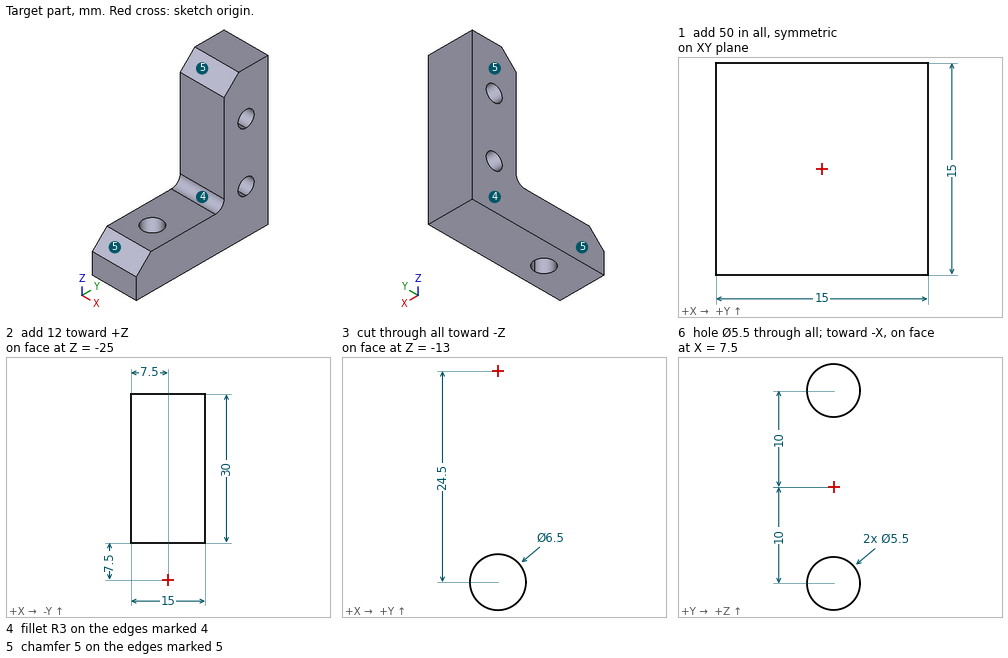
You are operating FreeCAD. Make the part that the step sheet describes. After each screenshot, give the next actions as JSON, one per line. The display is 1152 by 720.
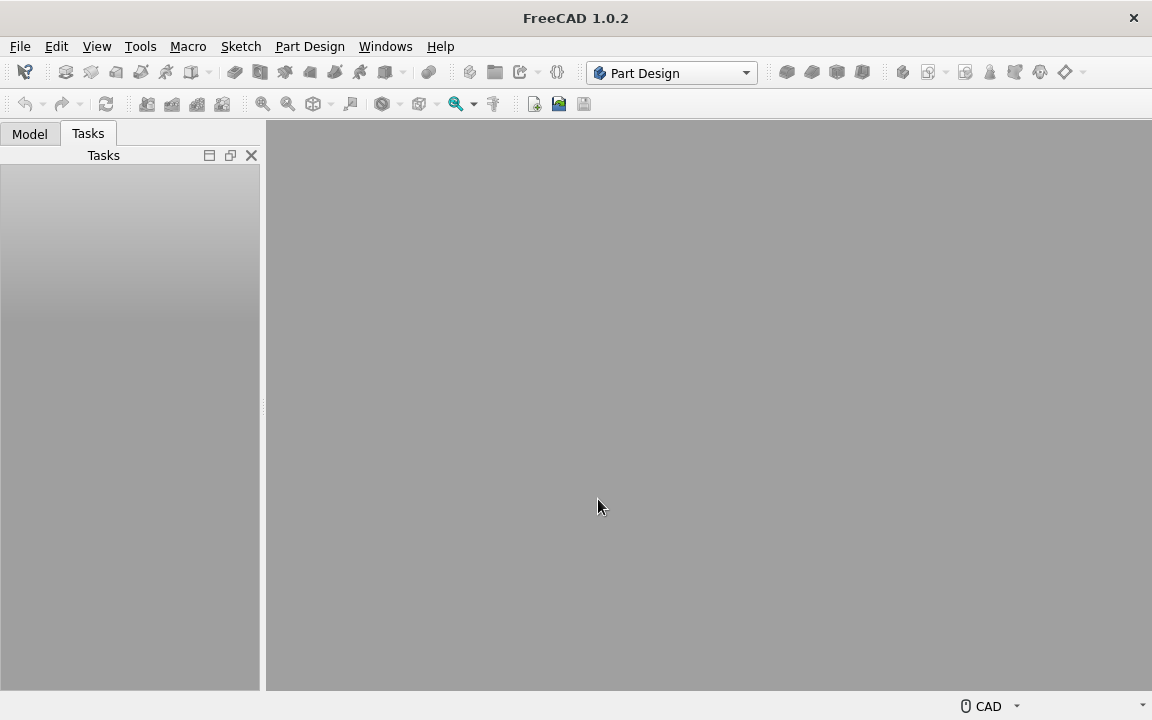
{"action": "left_click", "coordinate": [534, 104]}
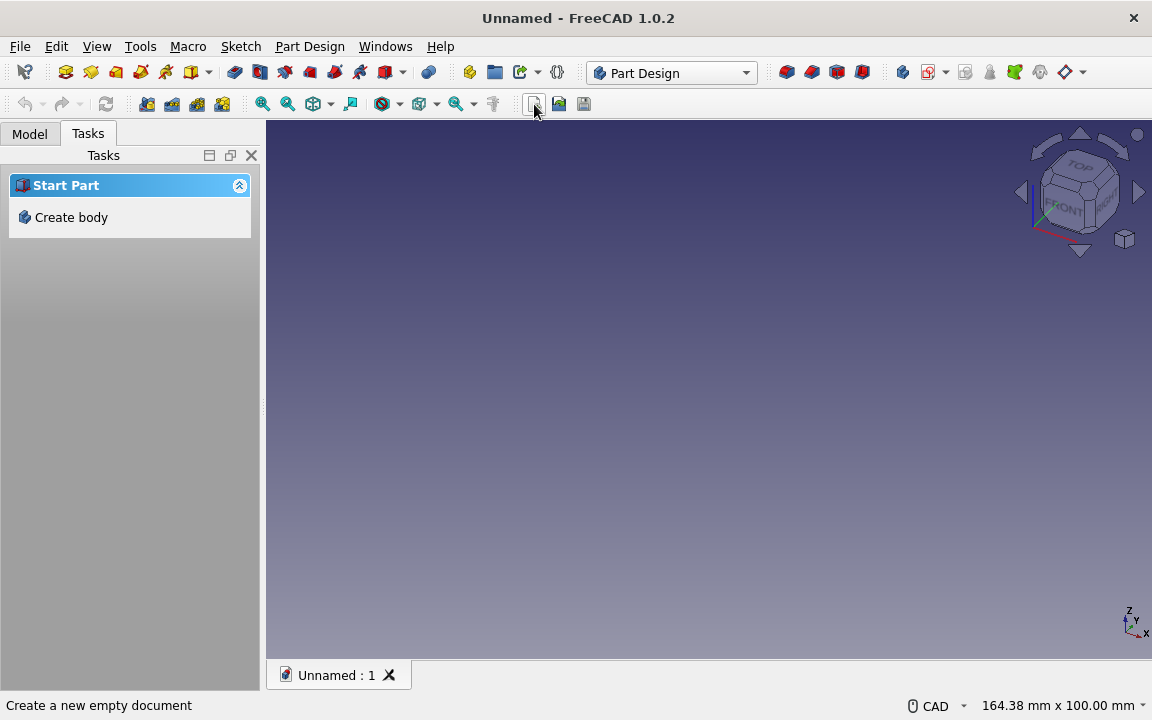
{"action": "left_click", "coordinate": [928, 72]}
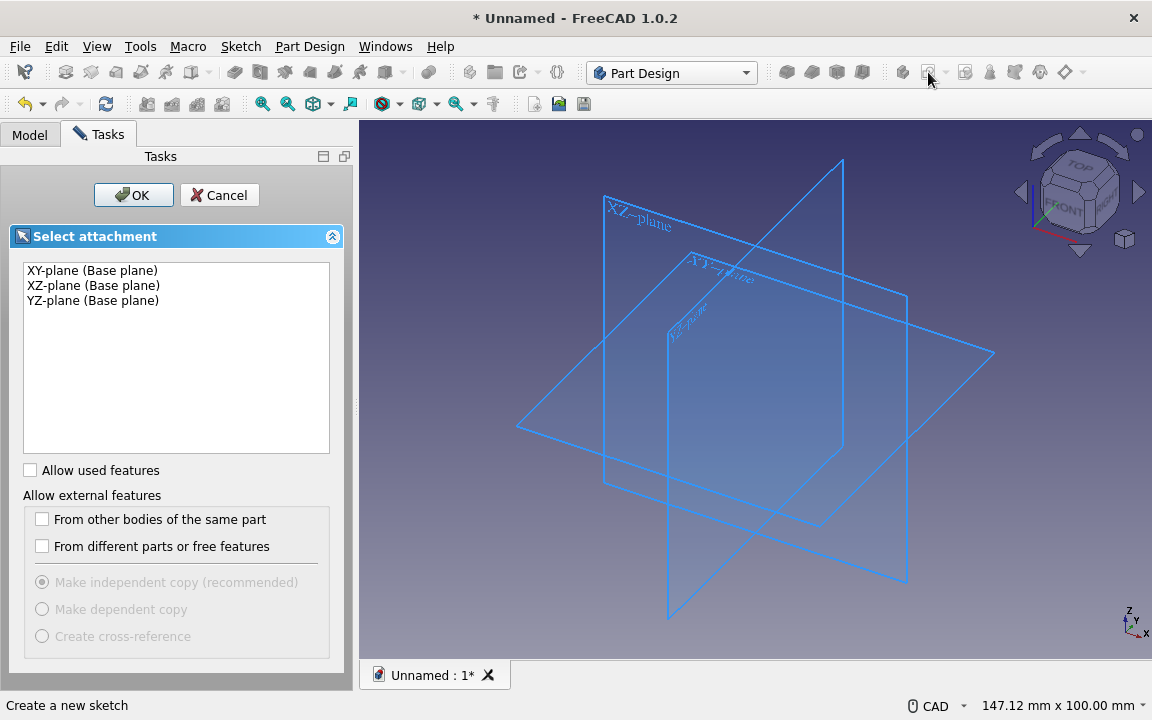
{"action": "left_click", "coordinate": [84, 270]}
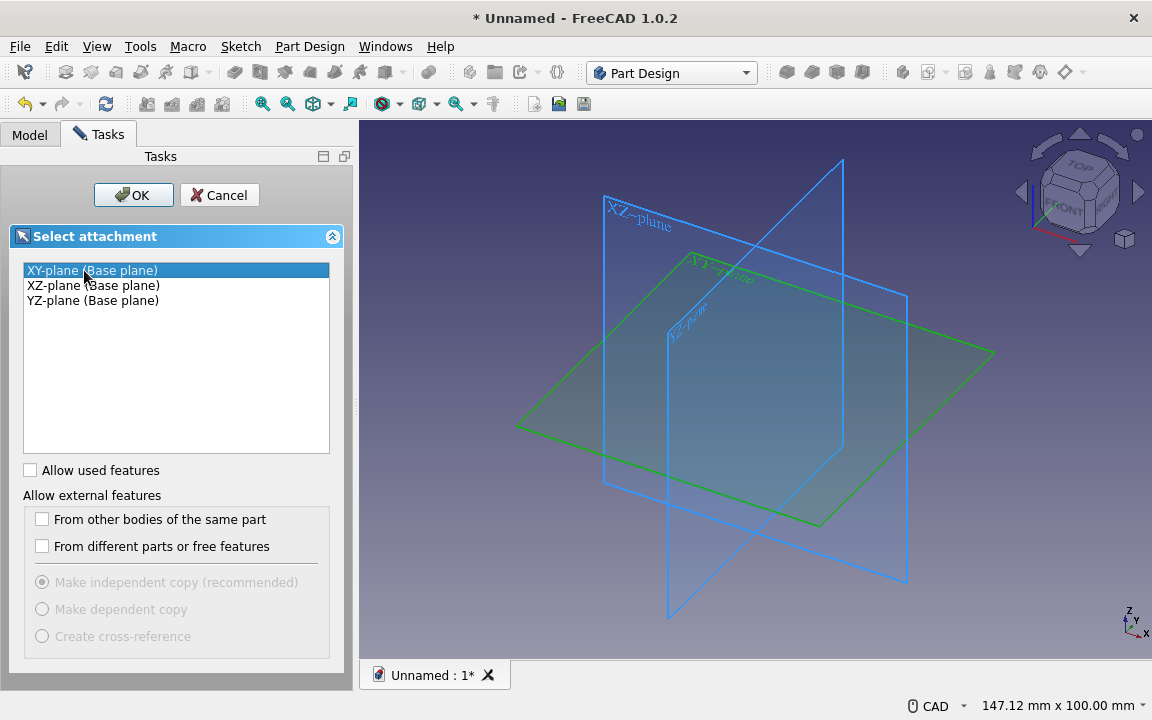
{"action": "left_click", "coordinate": [134, 195]}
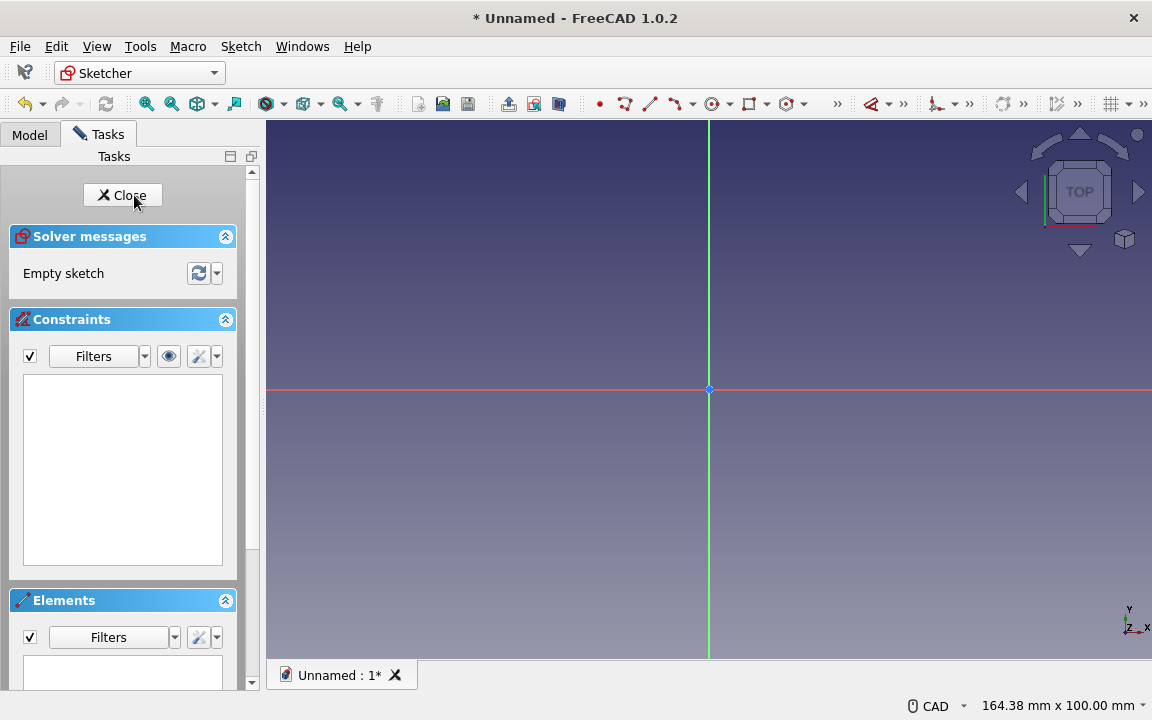
{"action": "scroll", "coordinate": [731, 390], "scroll_direction": "up", "scroll_amount": 7}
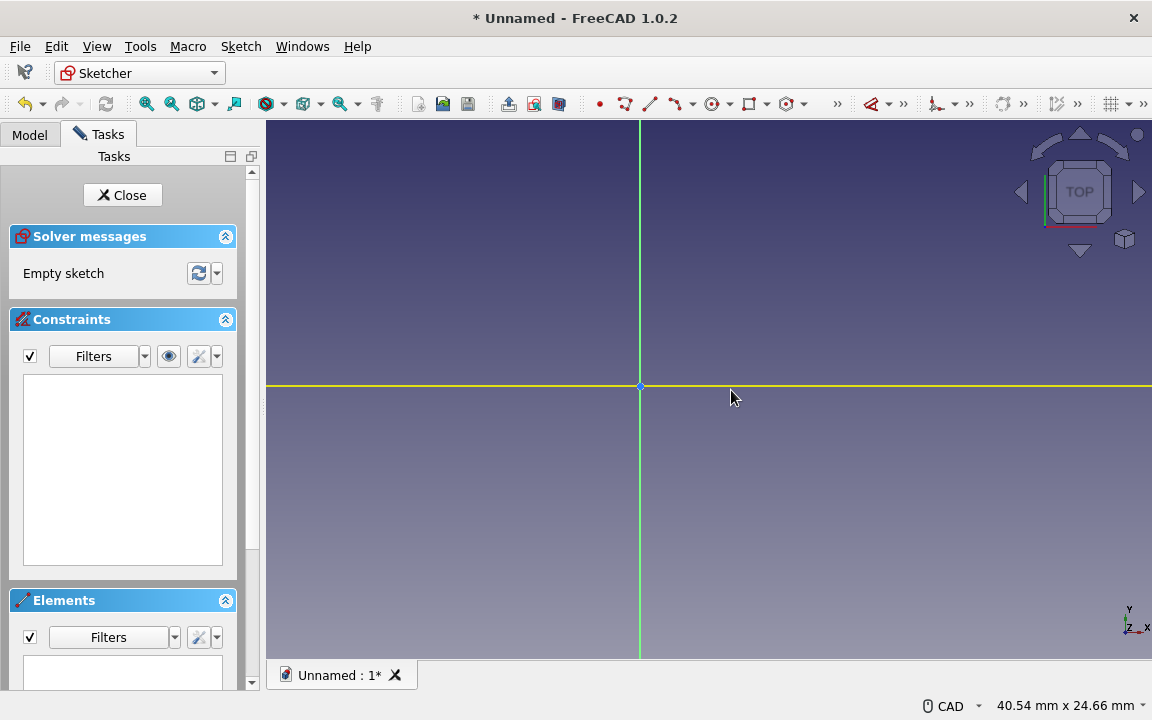
{"action": "key", "text": "g v"}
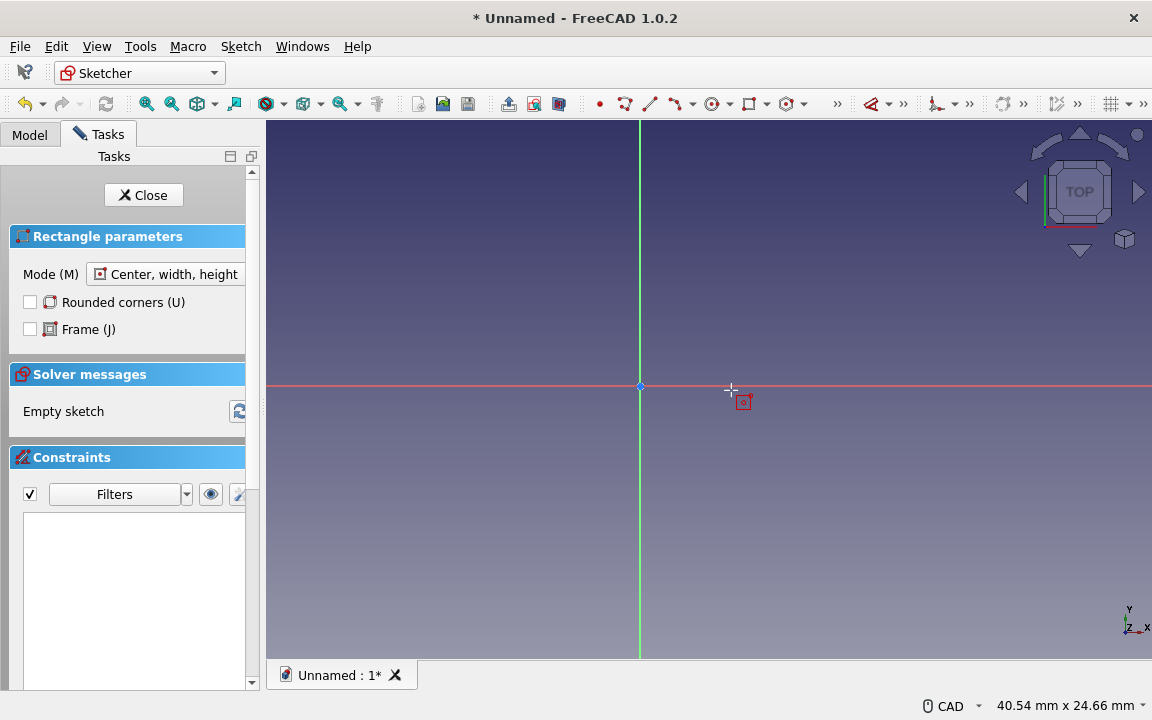
{"action": "left_click", "coordinate": [640, 386]}
{"action": "mouse_move", "coordinate": [804, 223]}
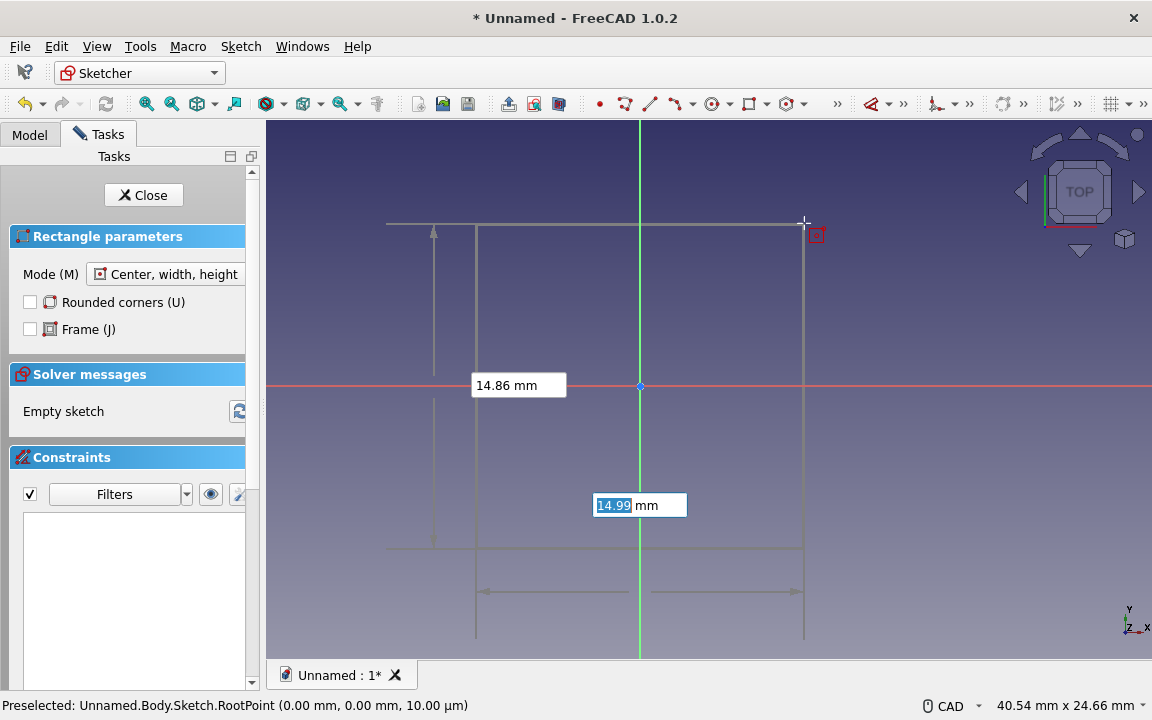
{"action": "type", "text": "15"}
{"action": "key", "text": "Tab"}
{"action": "type", "text": "15"}
{"action": "key", "text": "Return"}
{"action": "key", "text": "Escape"}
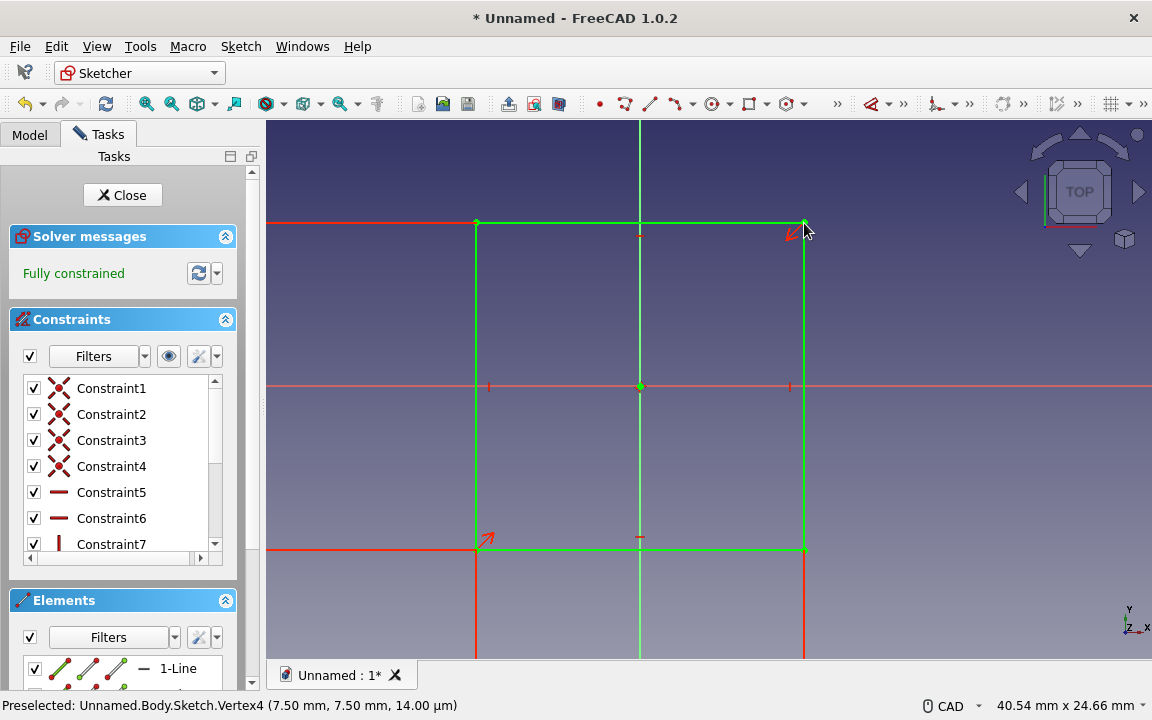
{"action": "left_click", "coordinate": [123, 195]}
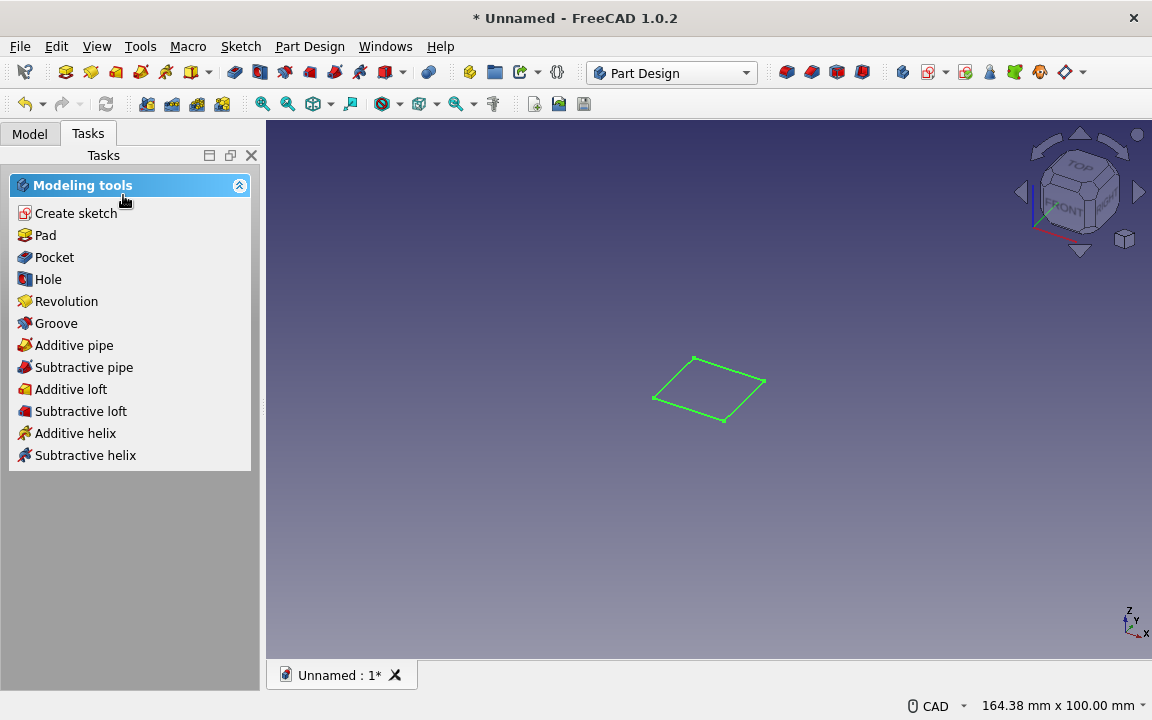
{"action": "left_click", "coordinate": [66, 72]}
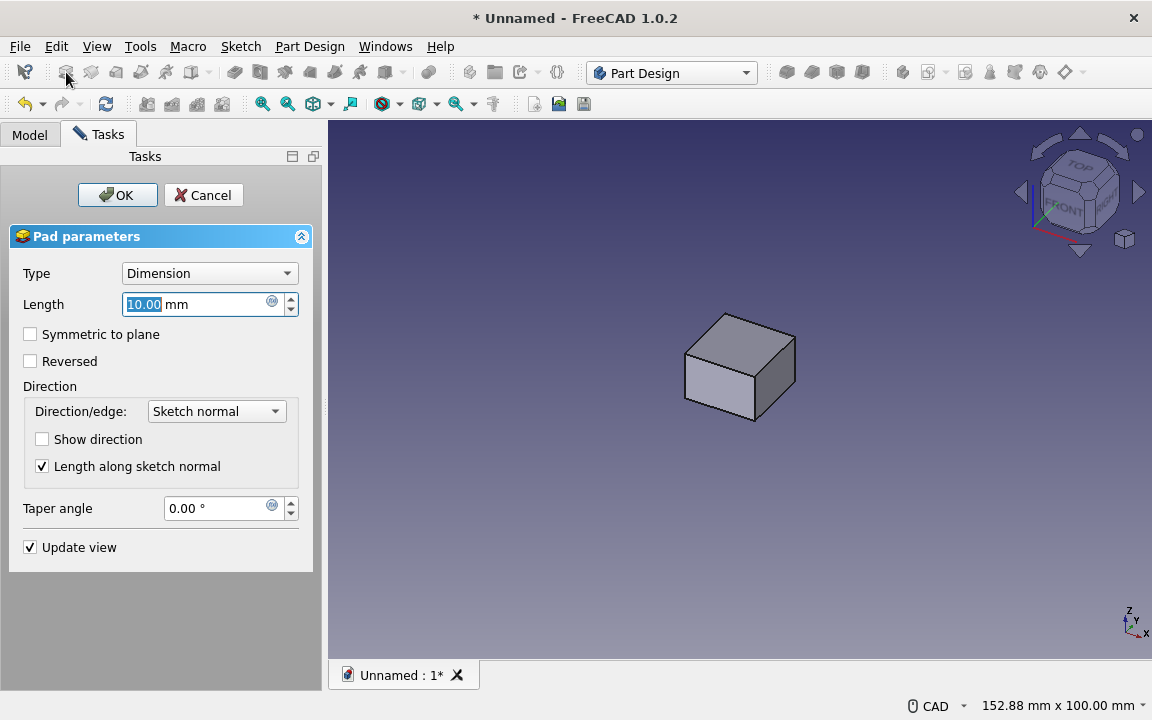
{"action": "type", "text": "50"}
{"action": "key", "text": "Tab"}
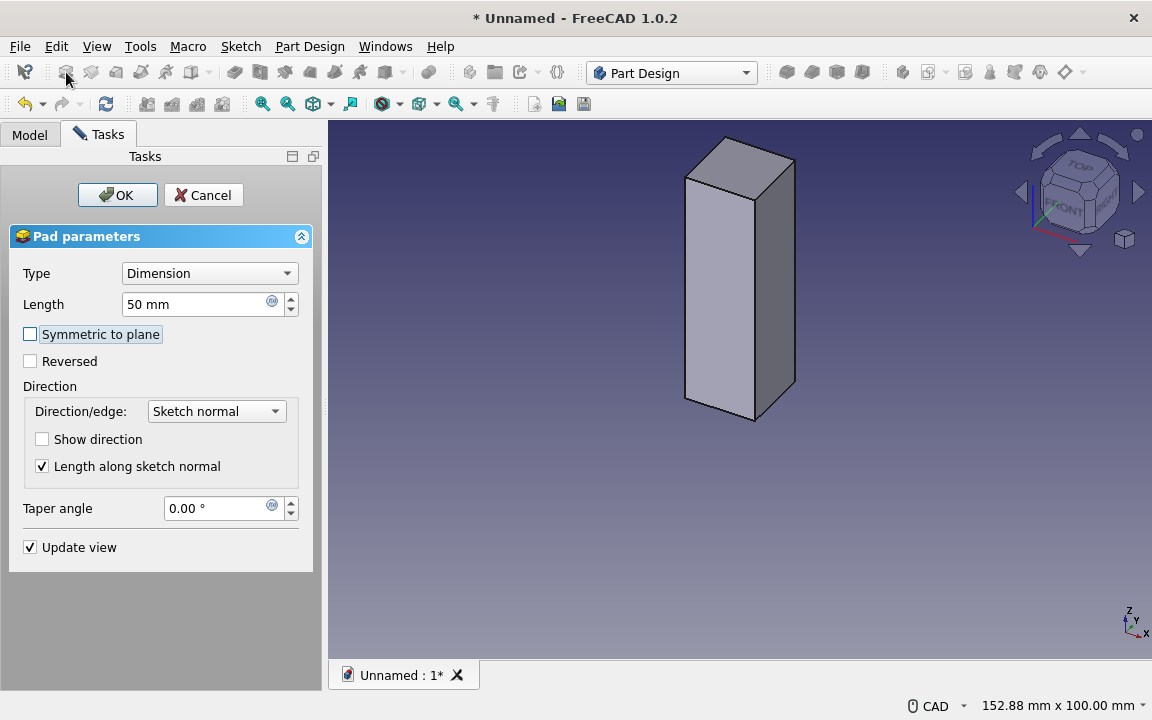
{"action": "left_click", "coordinate": [31, 334]}